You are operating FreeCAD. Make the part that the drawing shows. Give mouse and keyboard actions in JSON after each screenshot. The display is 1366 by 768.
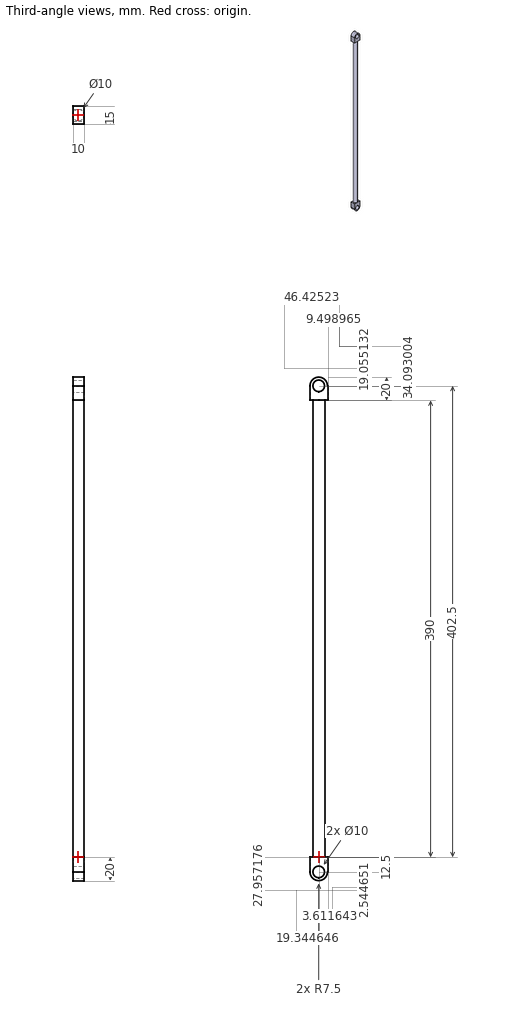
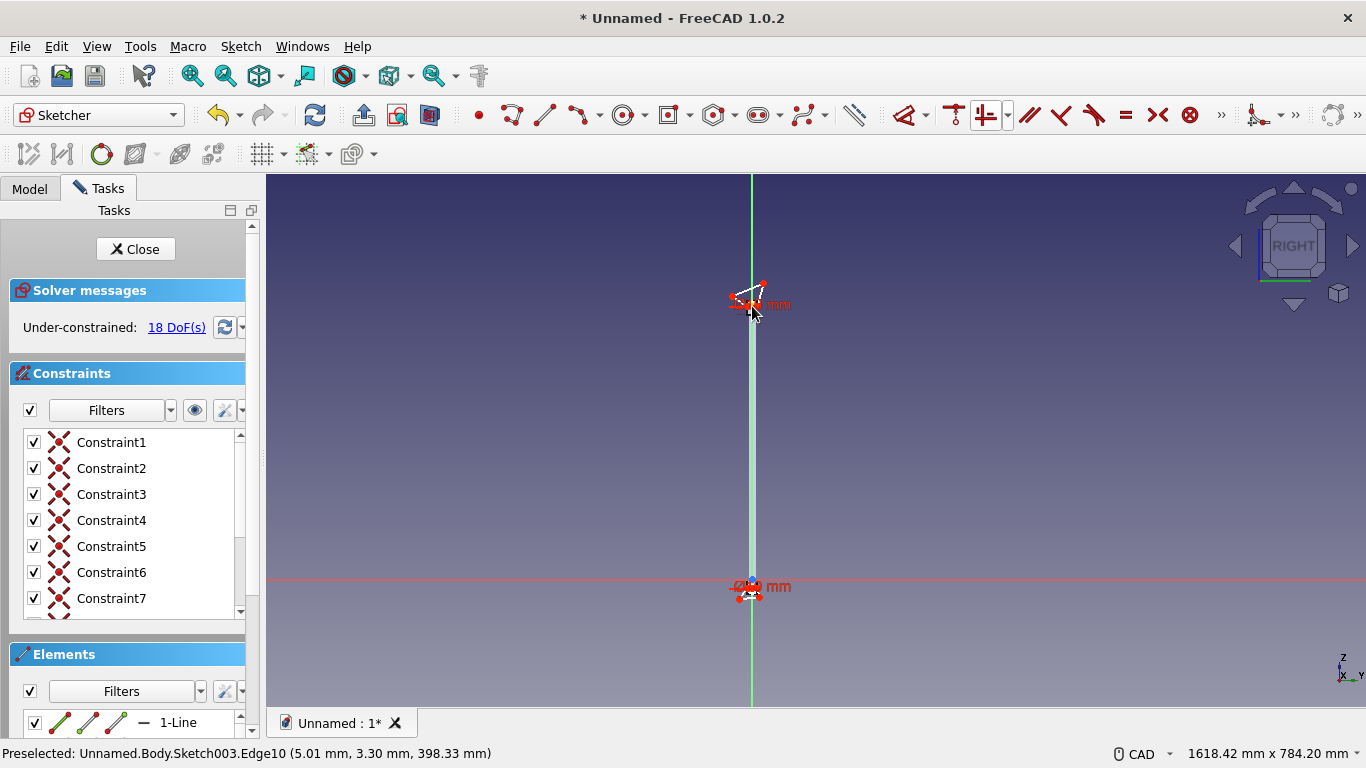
{"action": "scroll", "coordinate": [749, 593], "scroll_direction": "up", "scroll_amount": 11}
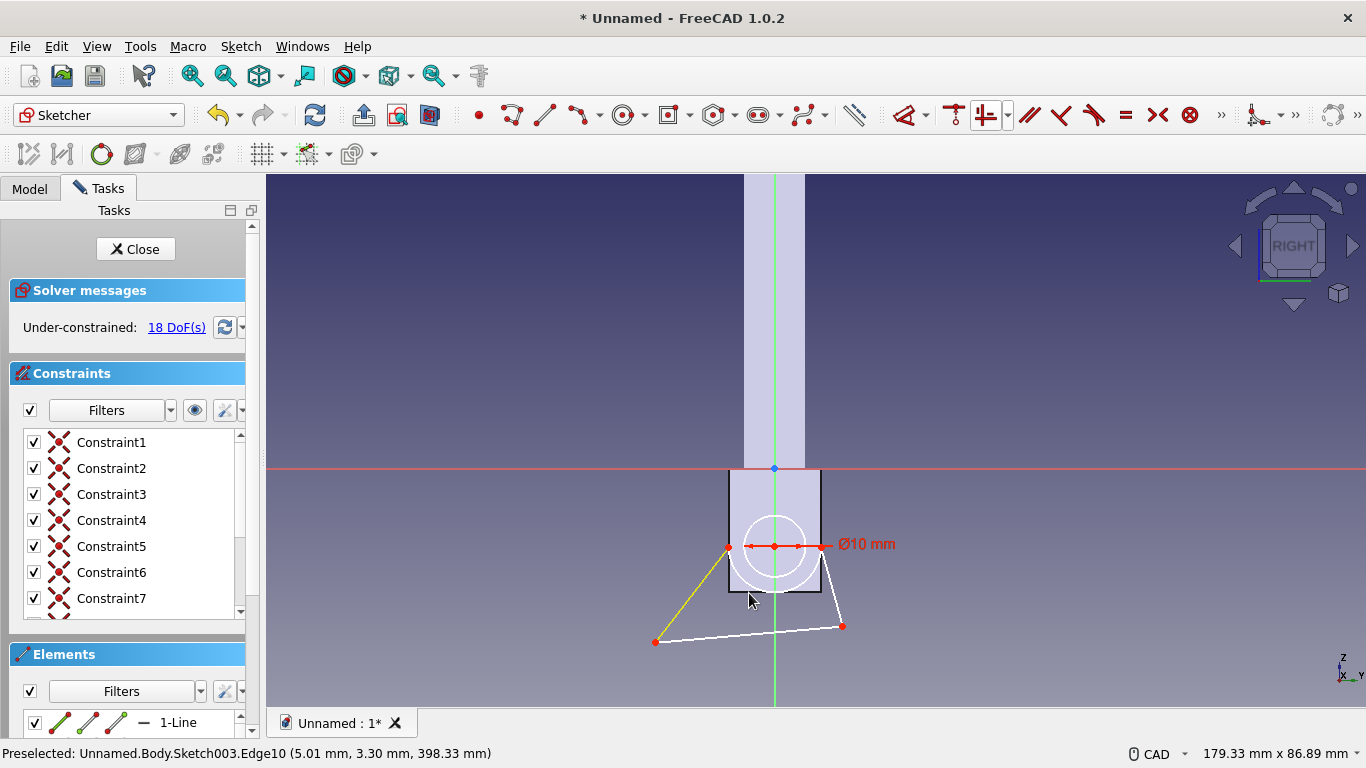
{"action": "left_click", "coordinate": [748, 584]}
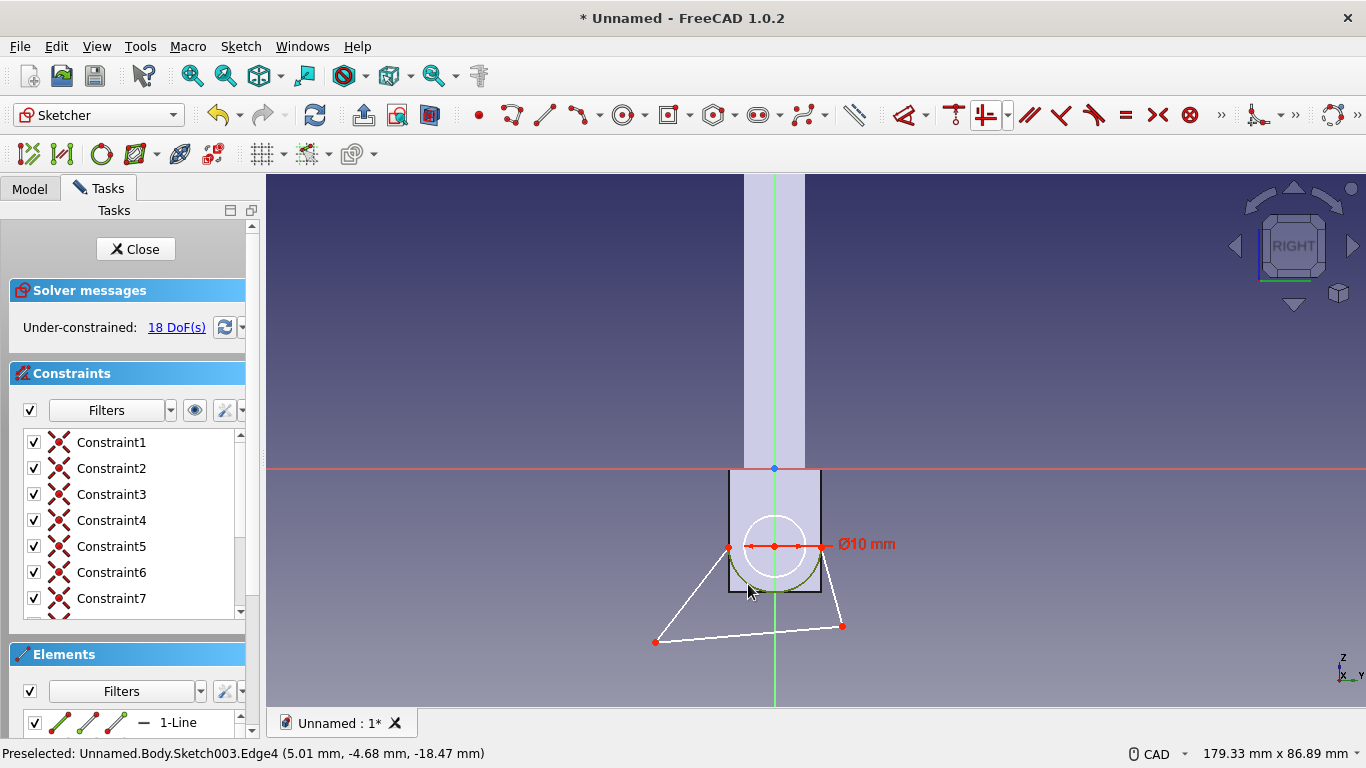
{"action": "scroll", "coordinate": [749, 593], "scroll_direction": "down", "scroll_amount": 11}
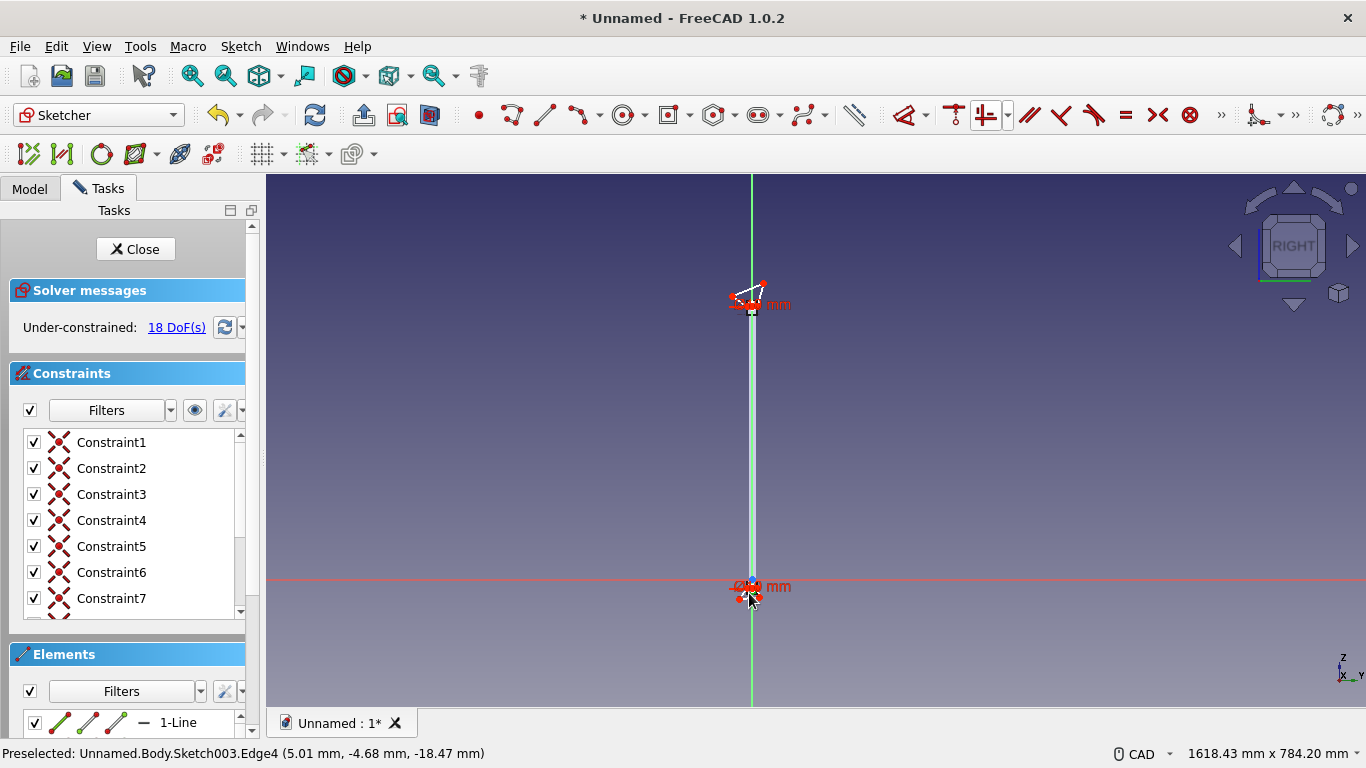
{"action": "scroll", "coordinate": [755, 302], "scroll_direction": "up", "scroll_amount": 11}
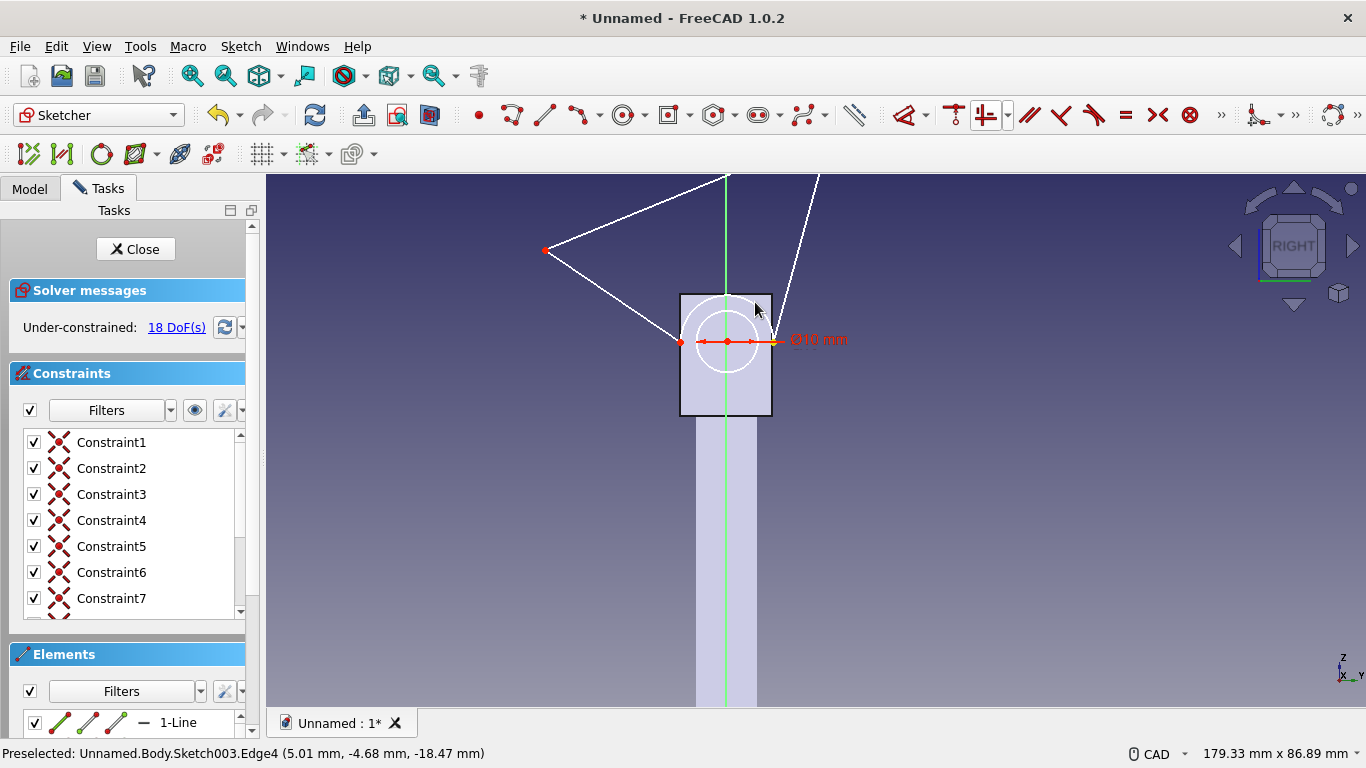
{"action": "left_click", "coordinate": [755, 304]}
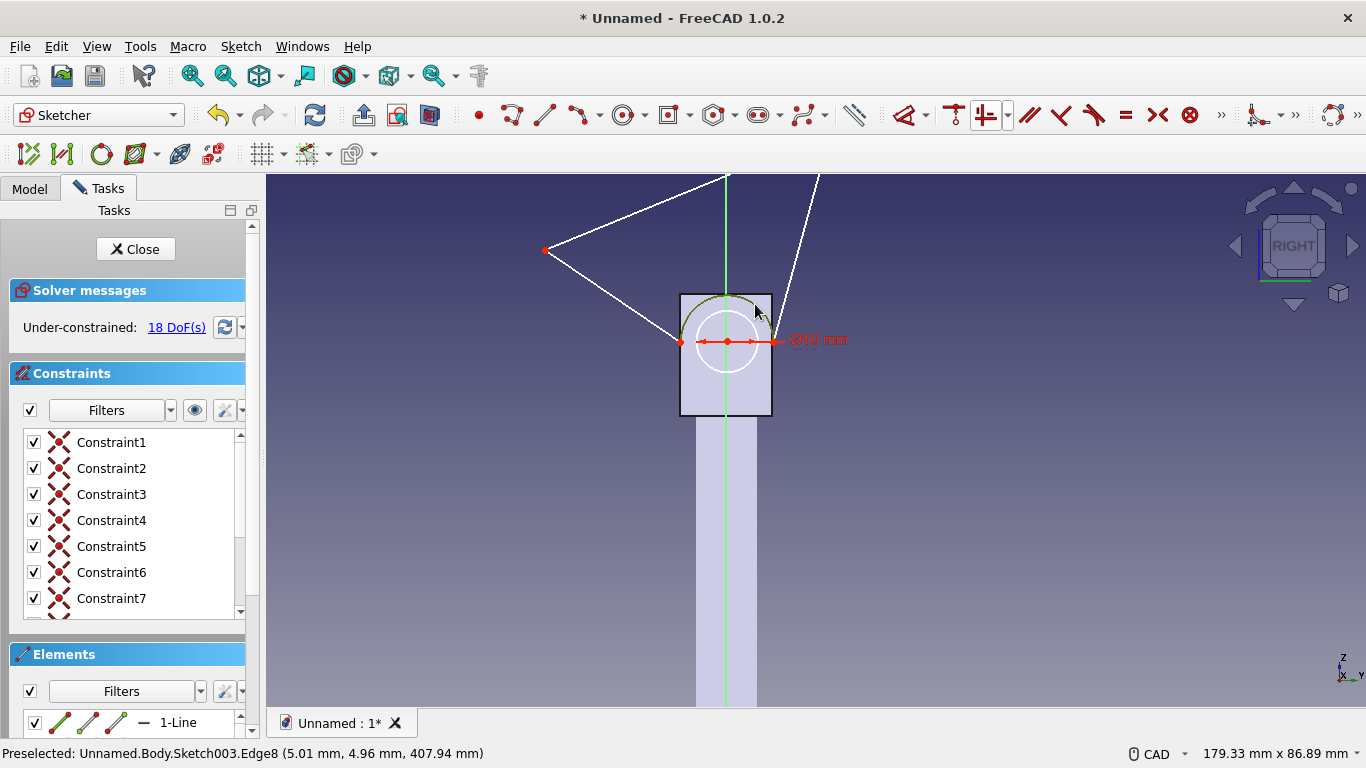
{"action": "left_click", "coordinate": [1126, 116]}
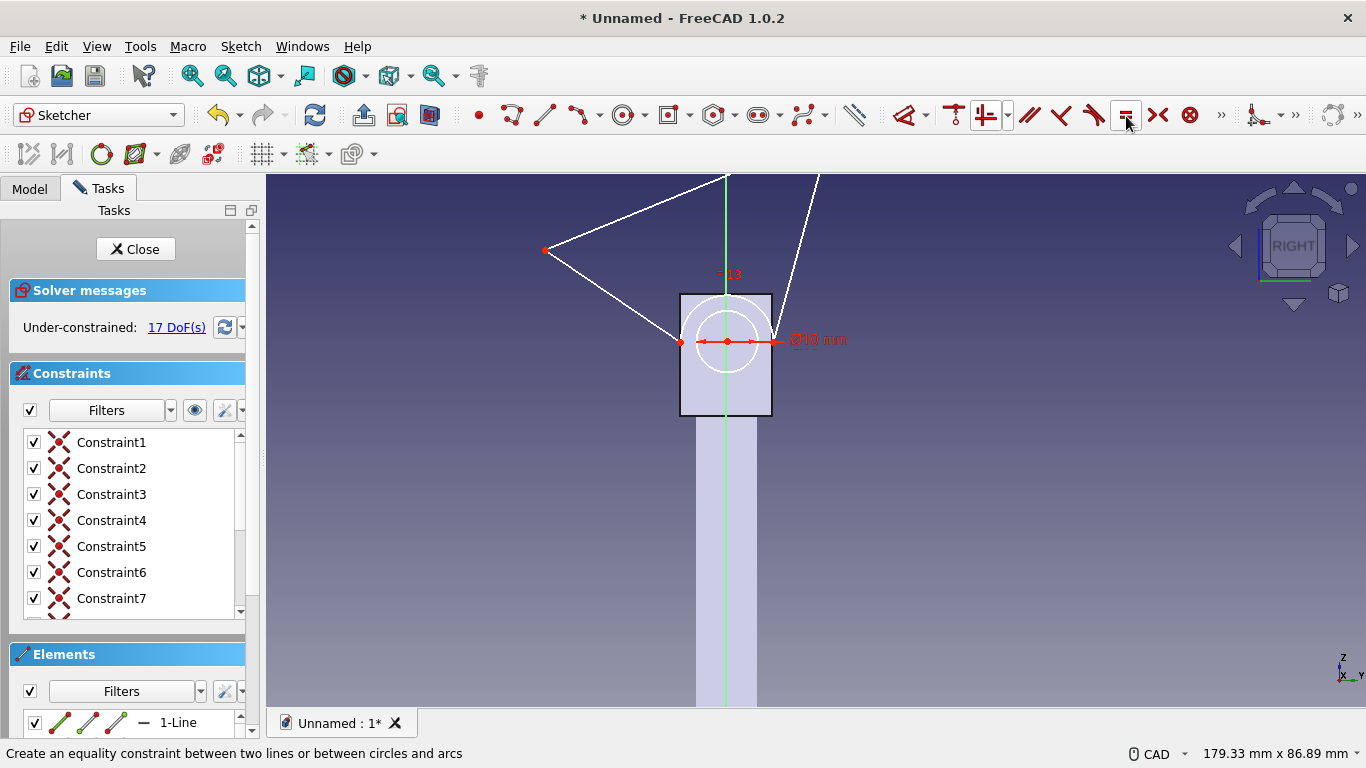
{"action": "scroll", "coordinate": [755, 302], "scroll_direction": "down", "scroll_amount": 11}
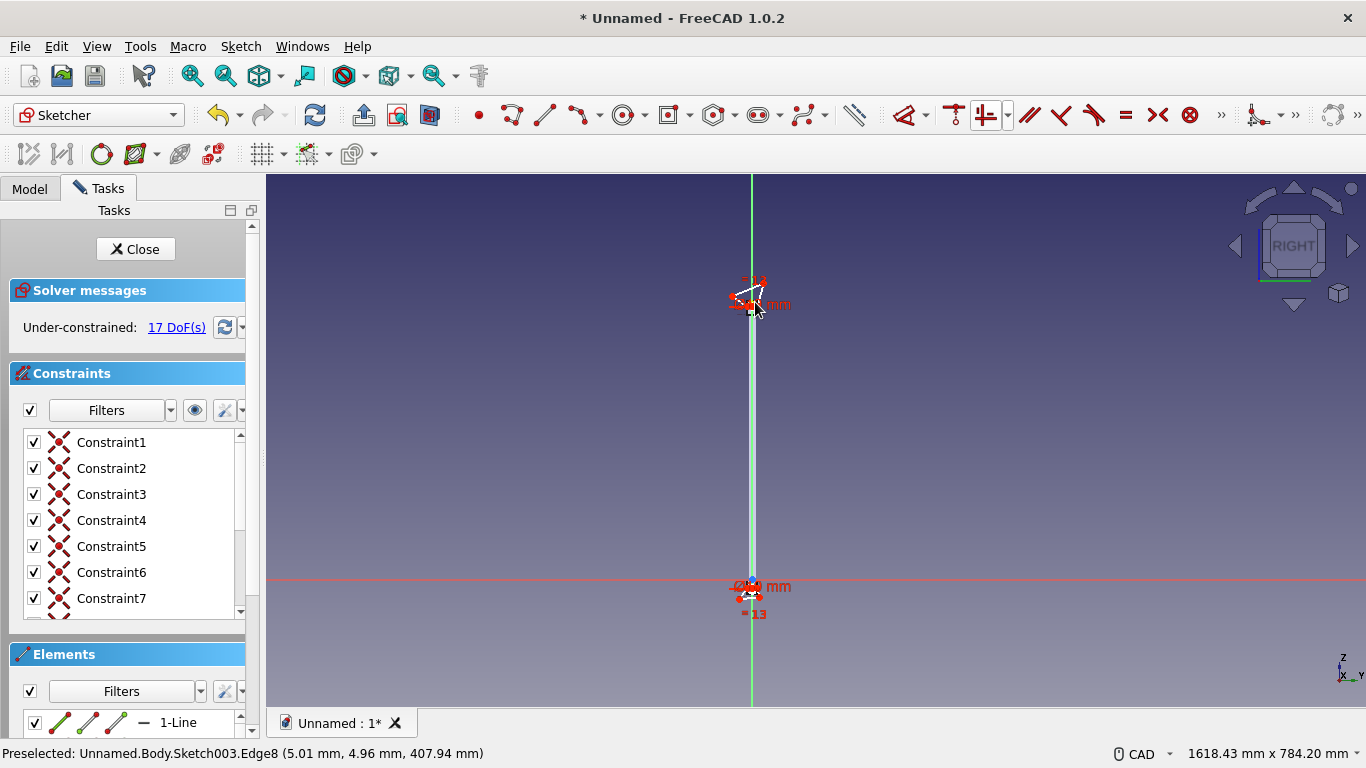
{"action": "scroll", "coordinate": [752, 589], "scroll_direction": "up", "scroll_amount": 5}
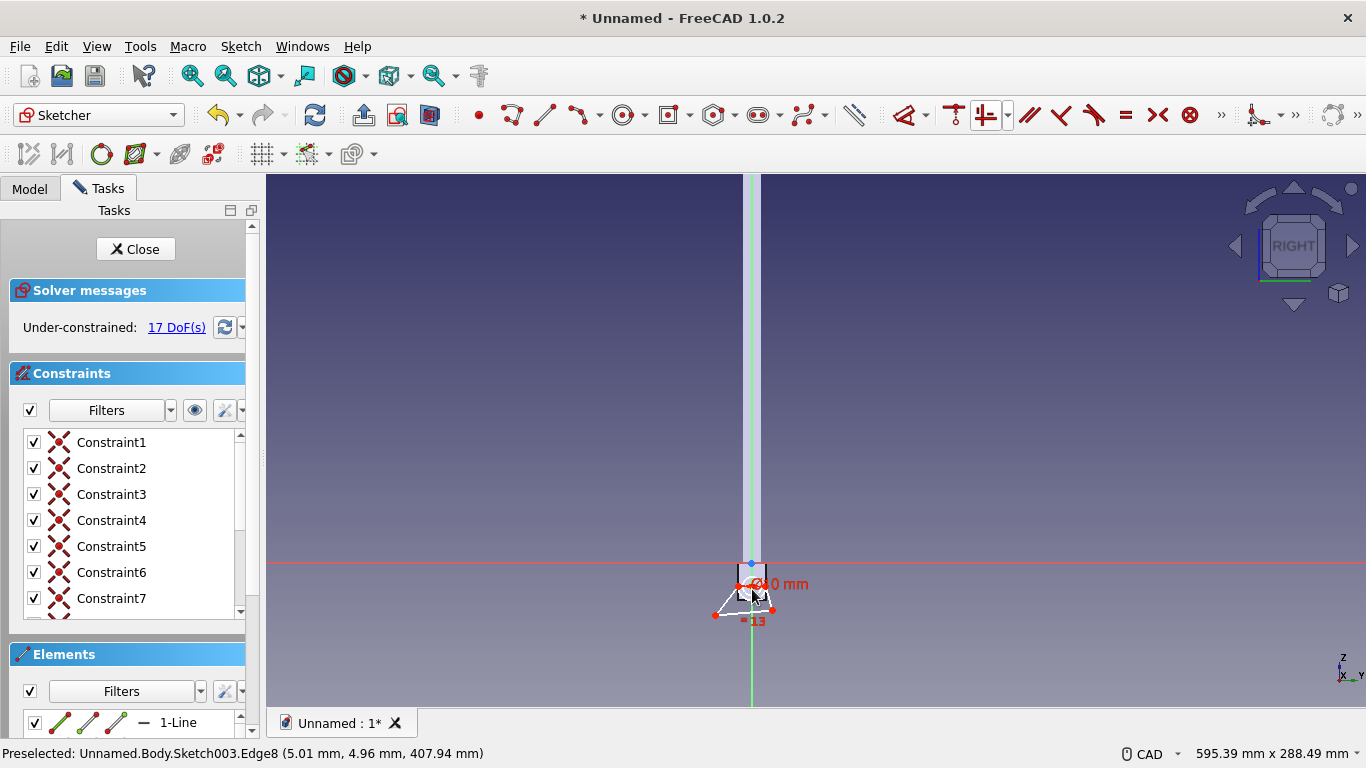
{"action": "left_click", "coordinate": [752, 586]}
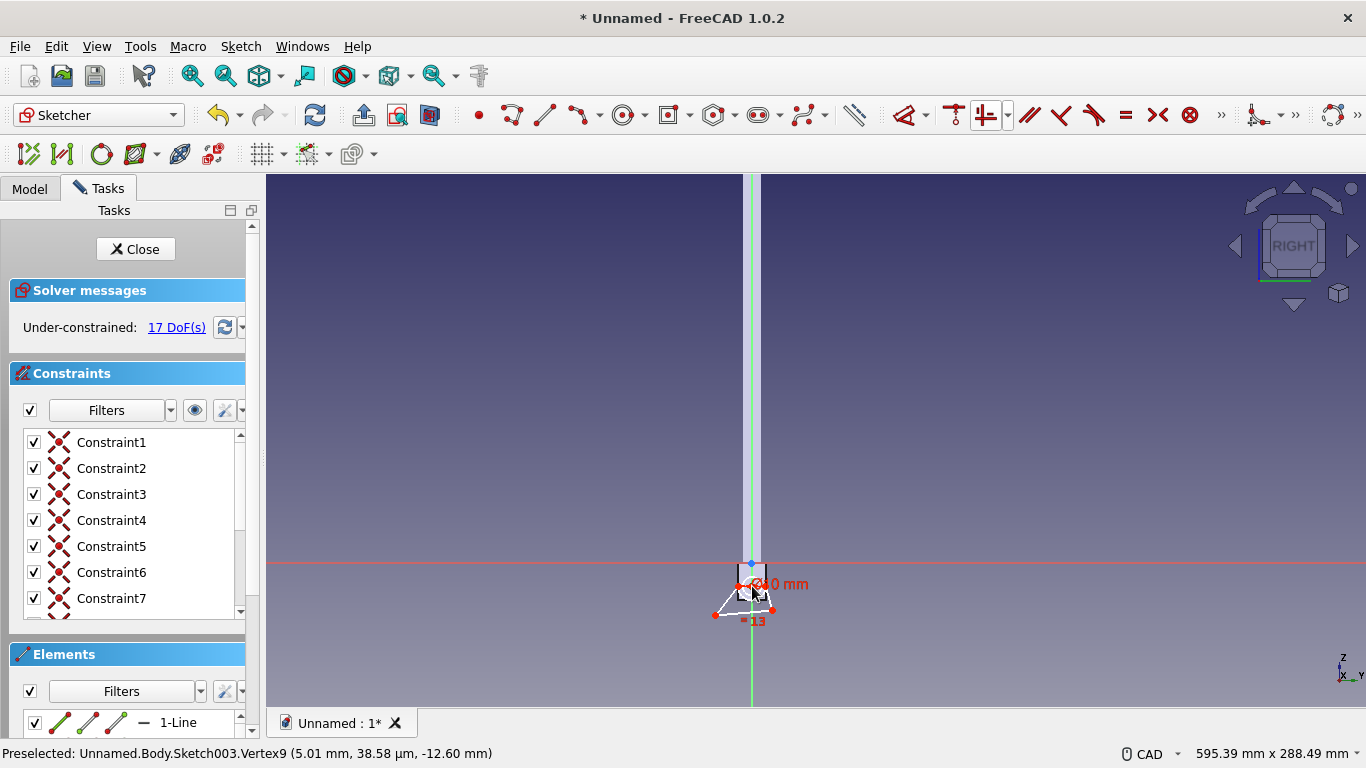
{"action": "left_click", "coordinate": [752, 645]}